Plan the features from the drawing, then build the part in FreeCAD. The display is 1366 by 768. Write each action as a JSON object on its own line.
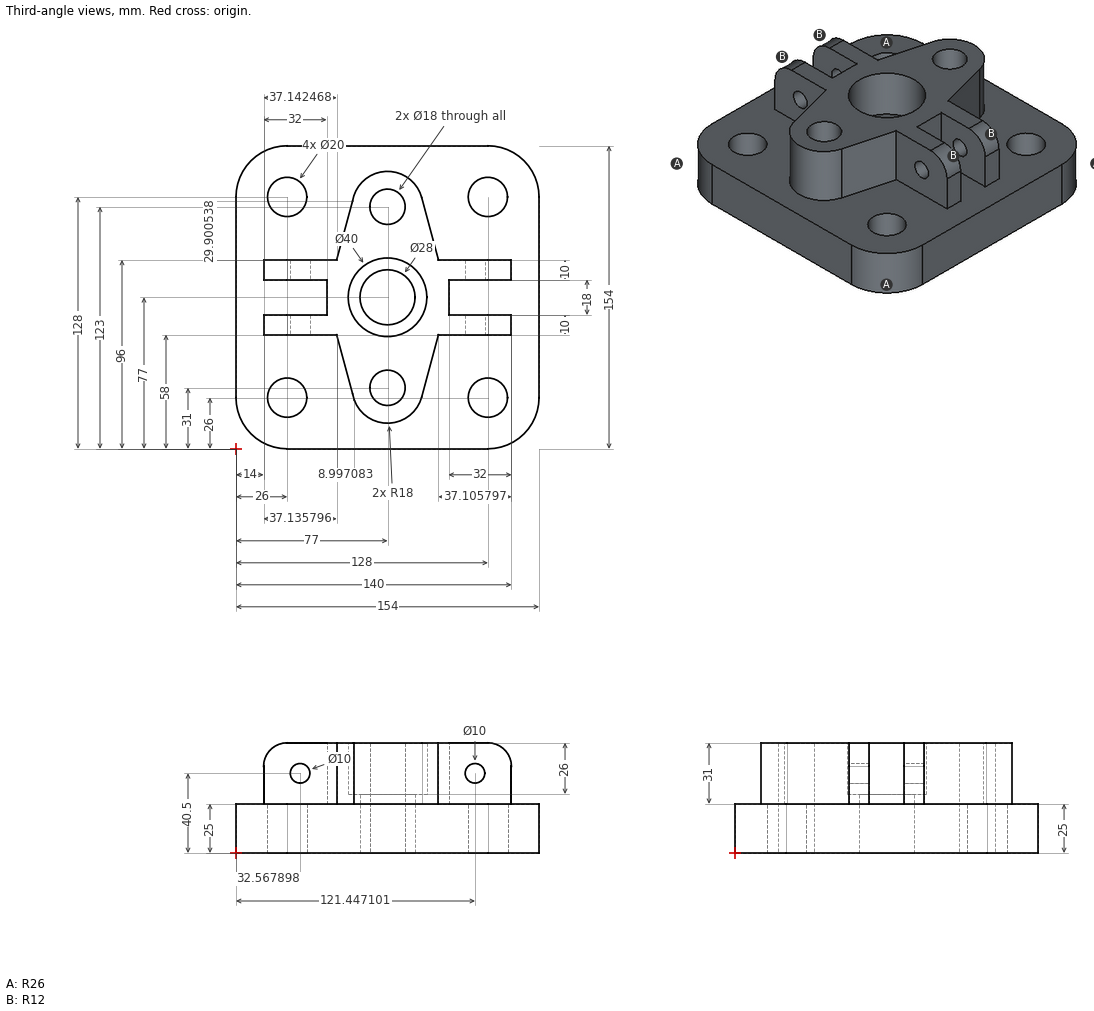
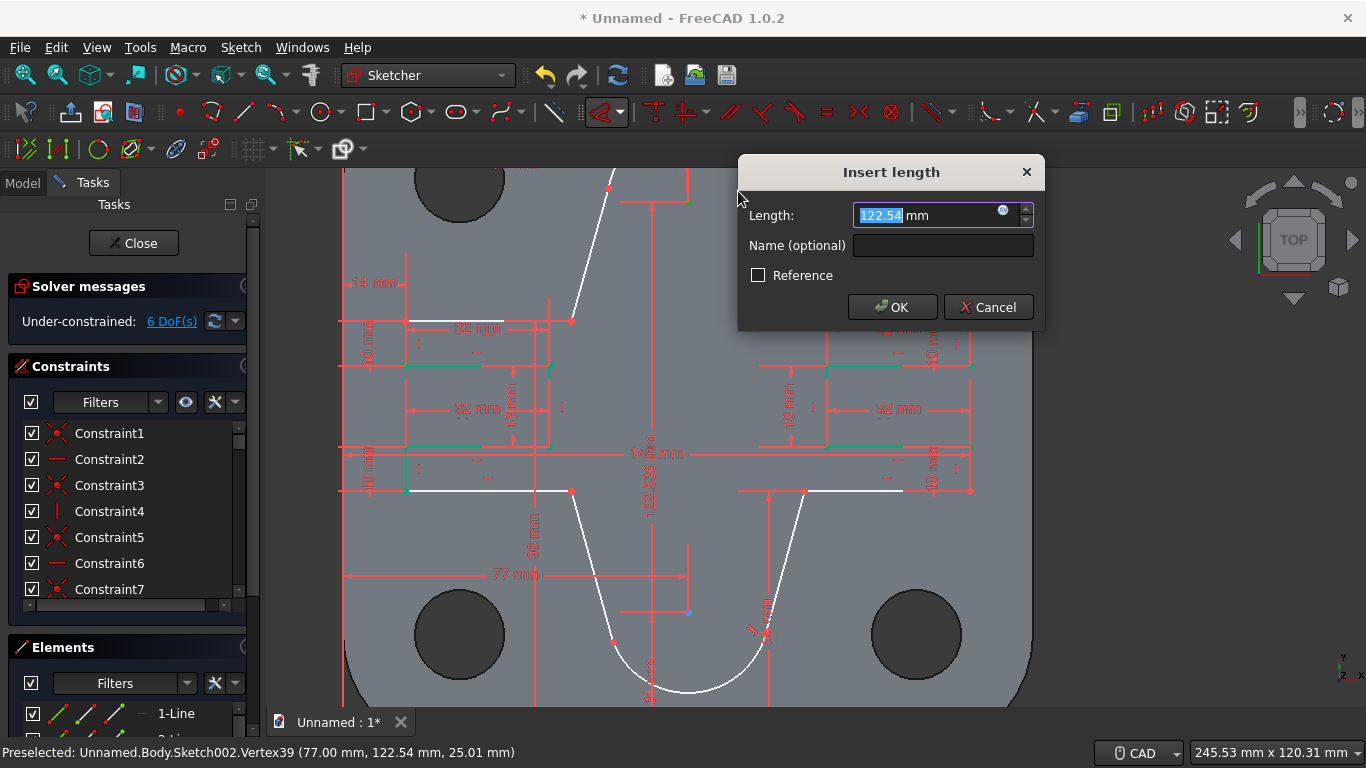
{"action": "type", "text": "123"}
{"action": "key", "text": "Return"}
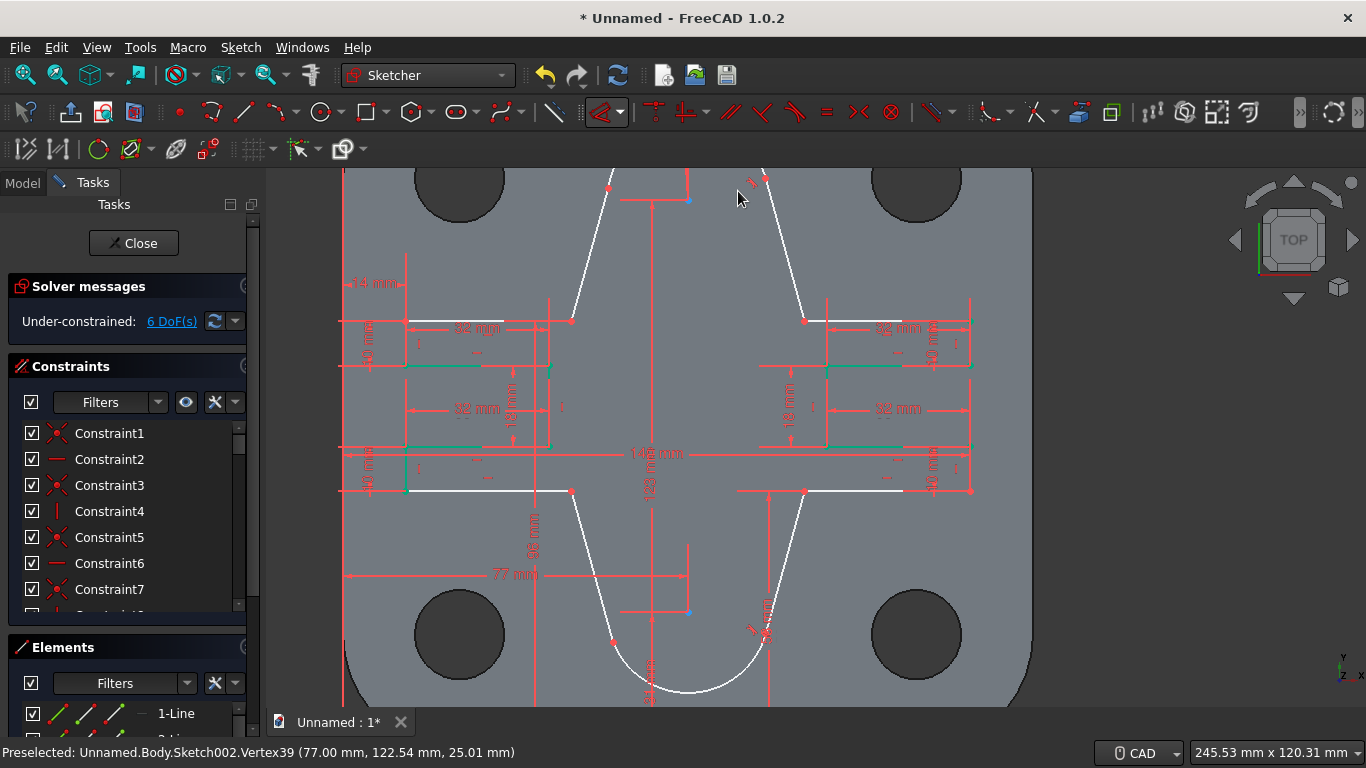
{"action": "left_click", "coordinate": [854, 491]}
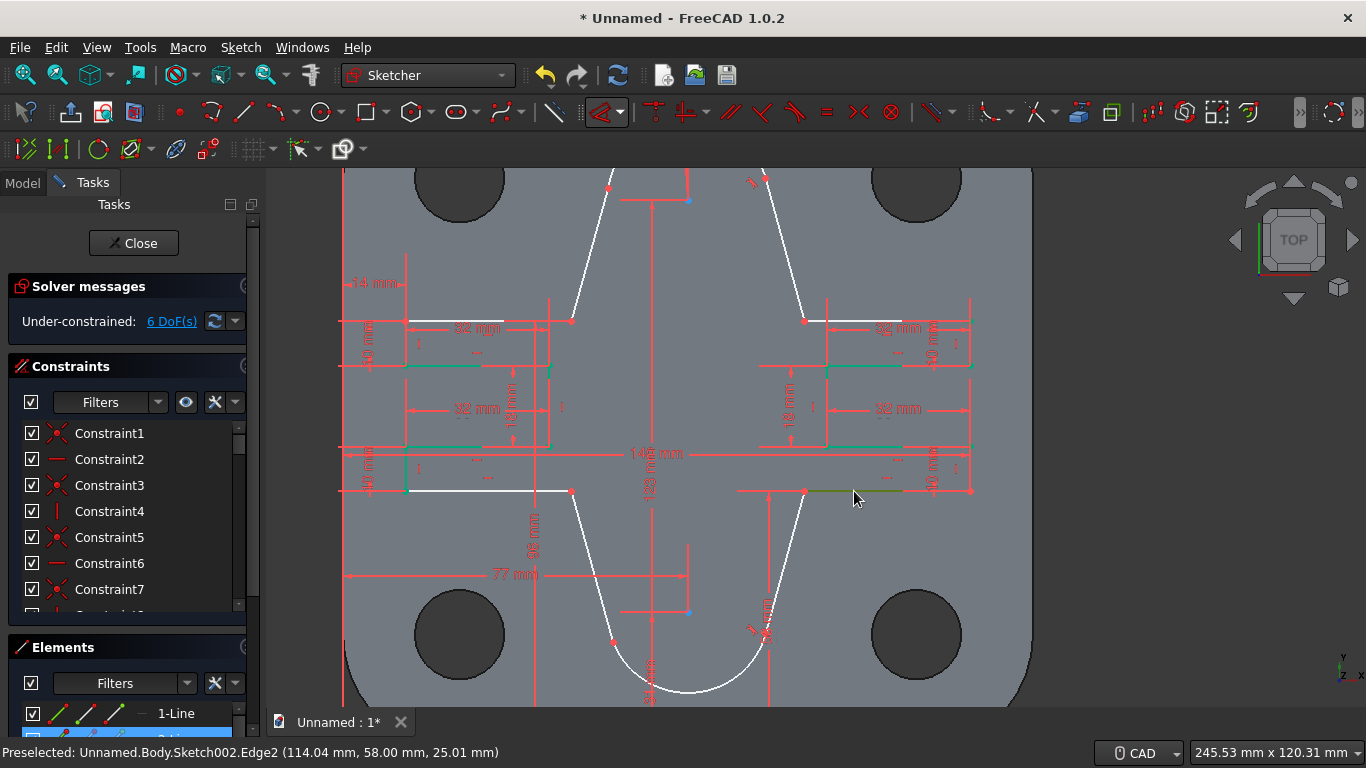
{"action": "left_click", "coordinate": [622, 112]}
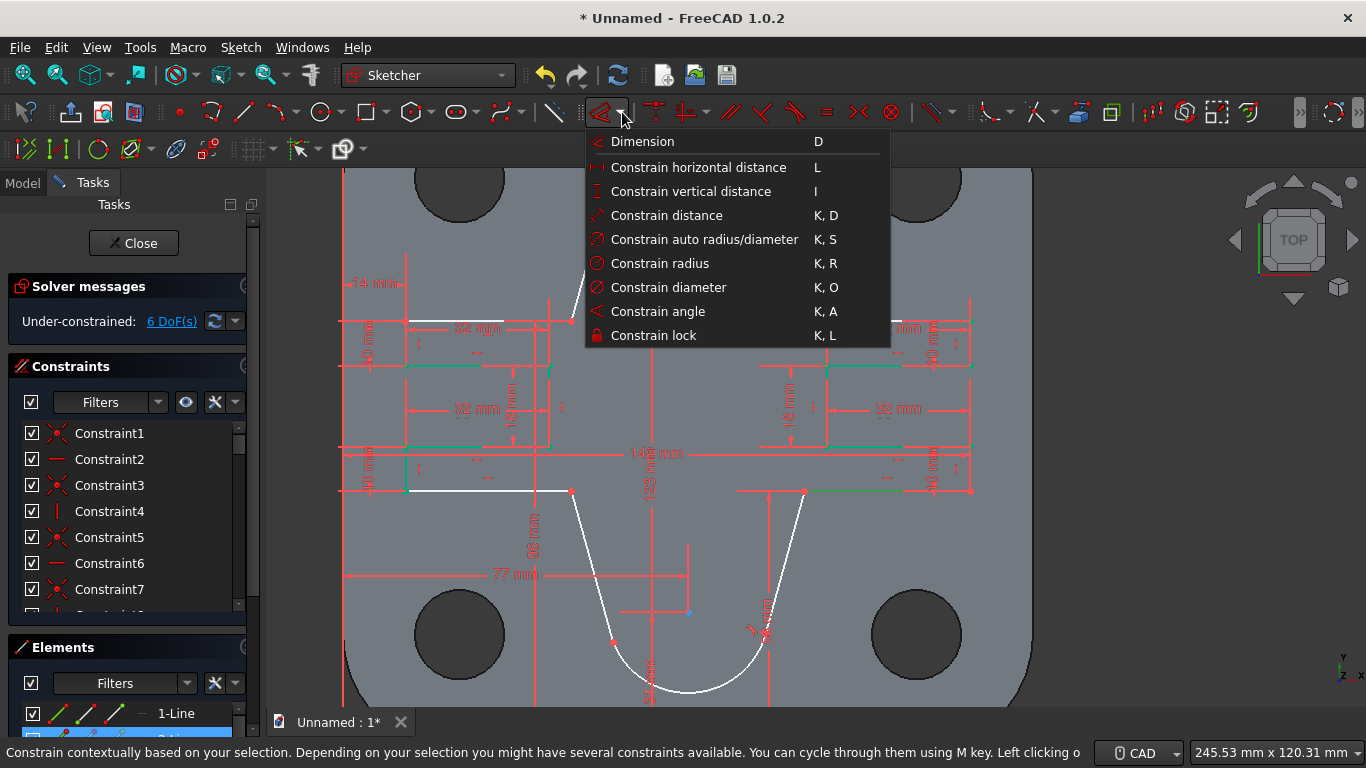
{"action": "left_click", "coordinate": [738, 167]}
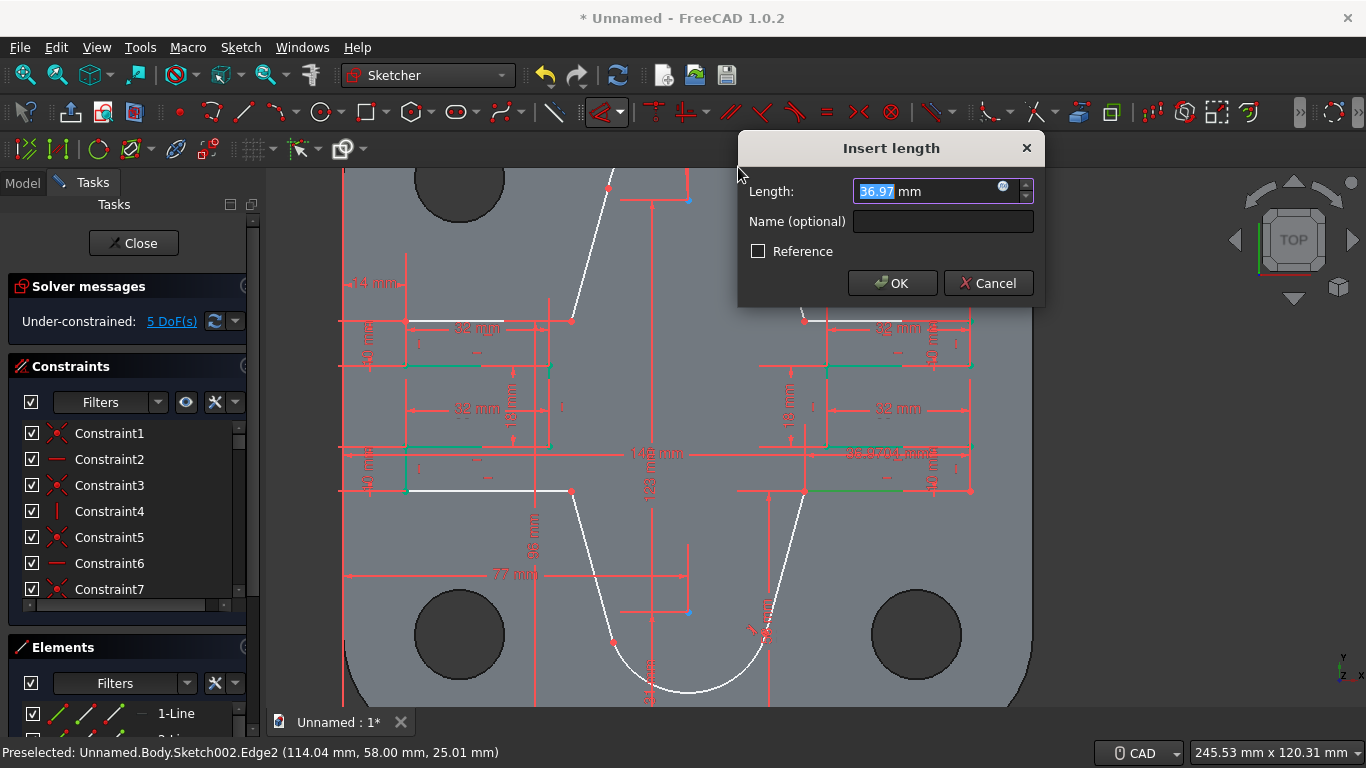
{"action": "type", "text": "37.105797"}
{"action": "key", "text": "Return"}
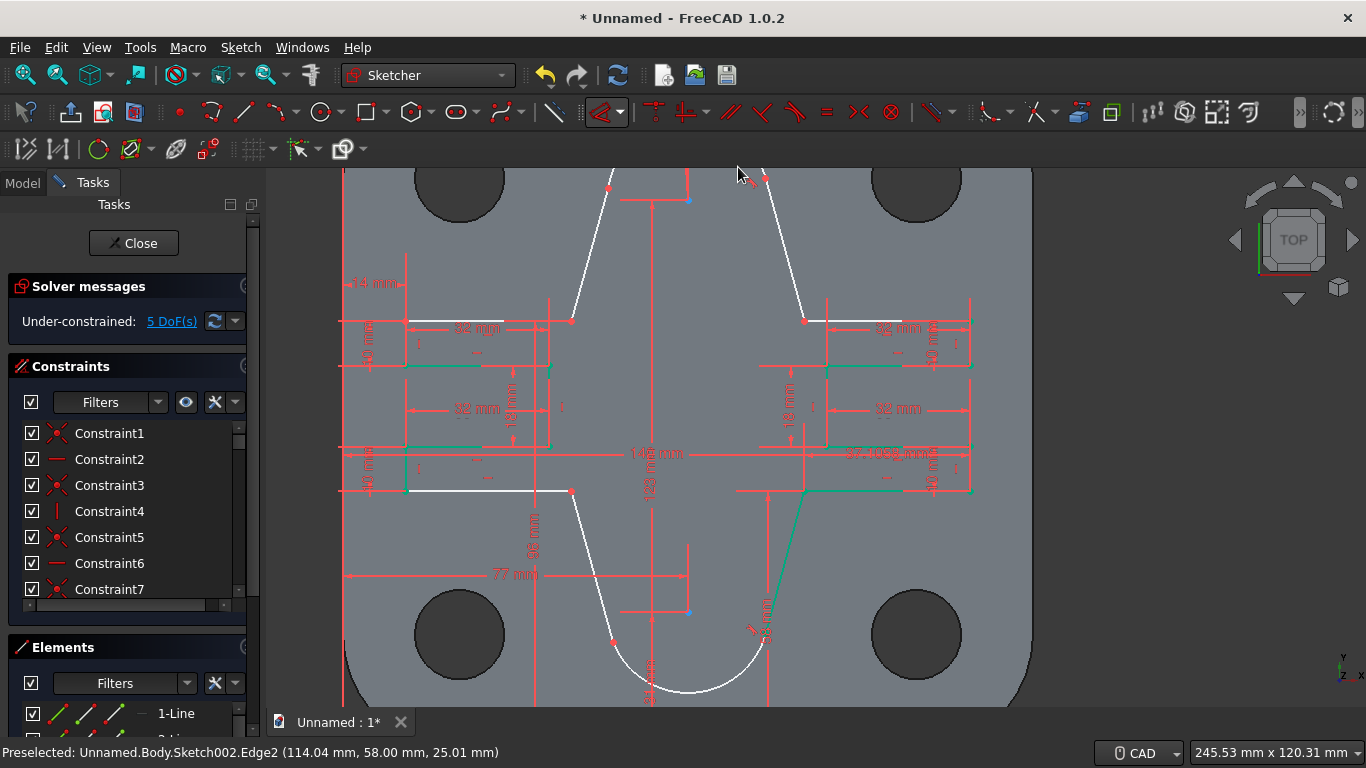
{"action": "left_click", "coordinate": [854, 321]}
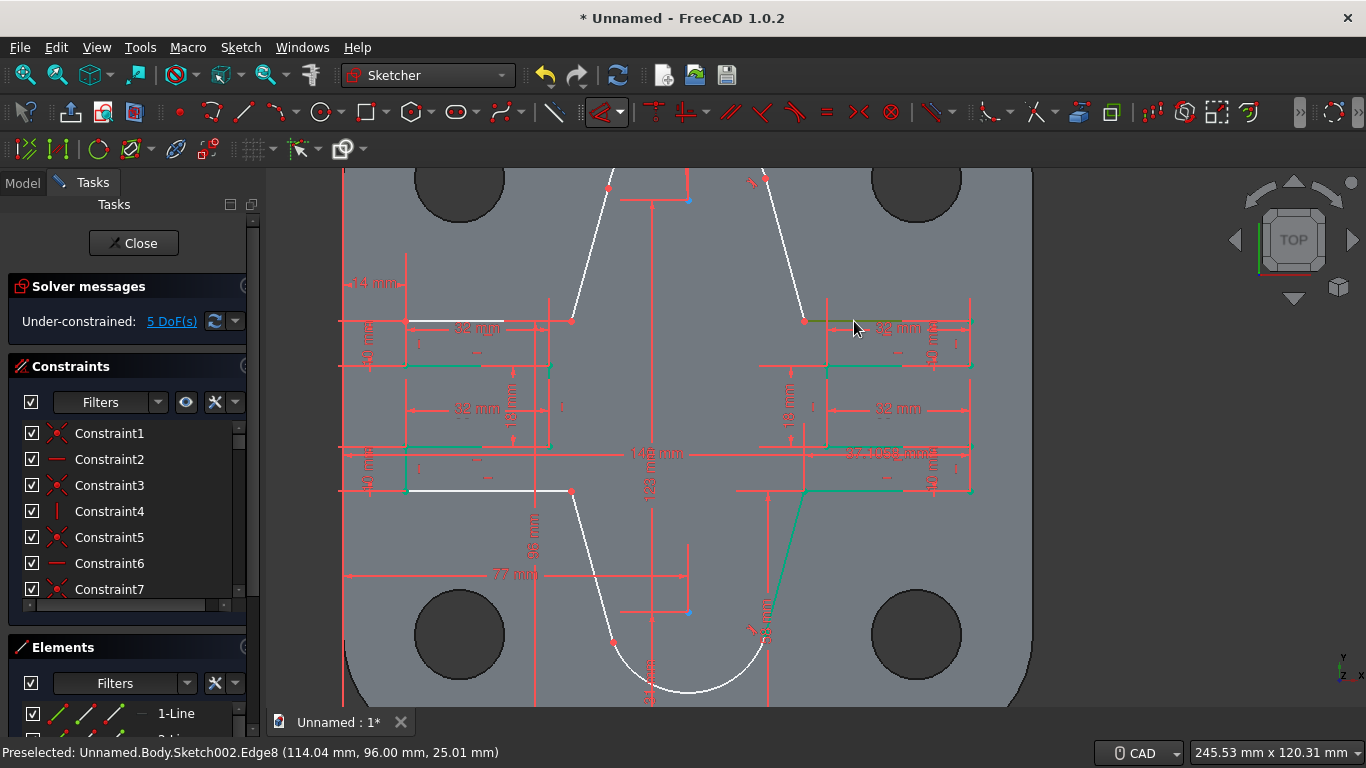
{"action": "key", "text": "l"}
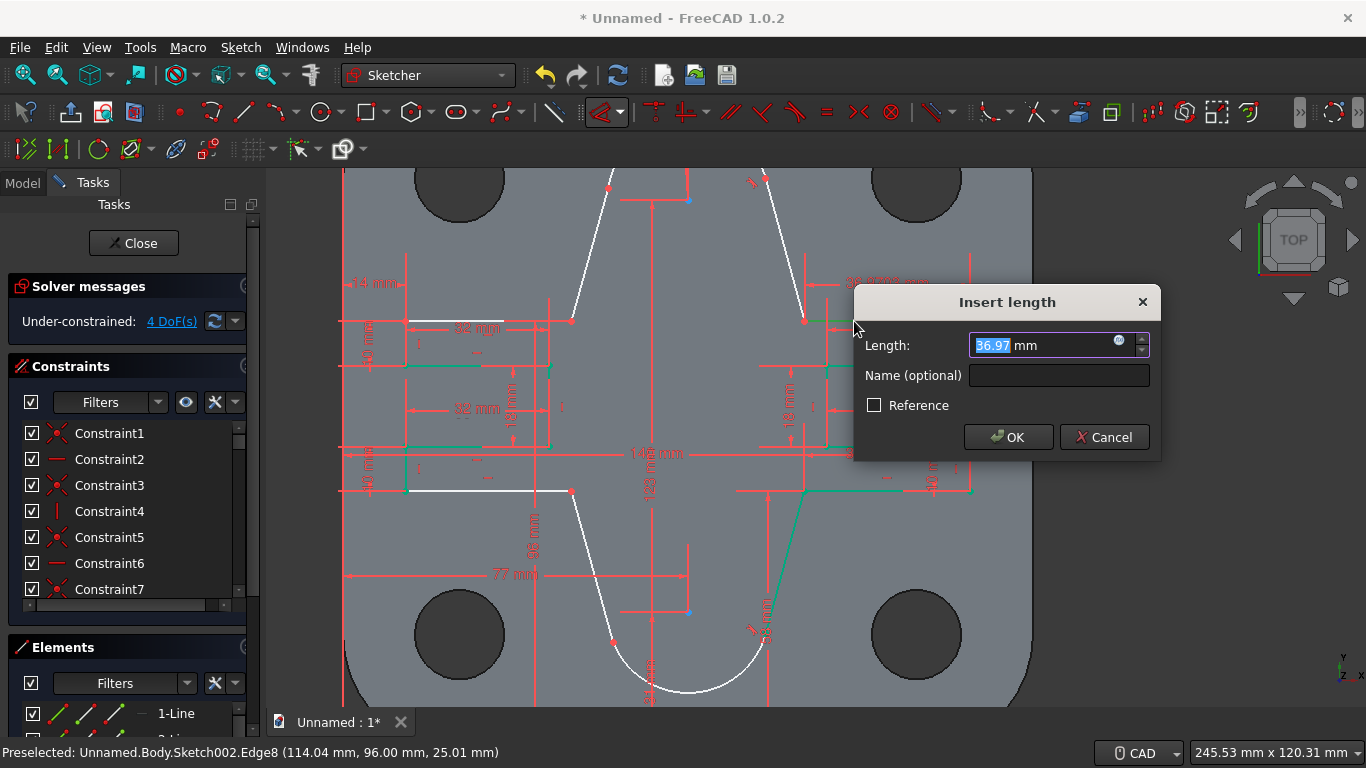
{"action": "type", "text": "37.105797"}
{"action": "key", "text": "Return"}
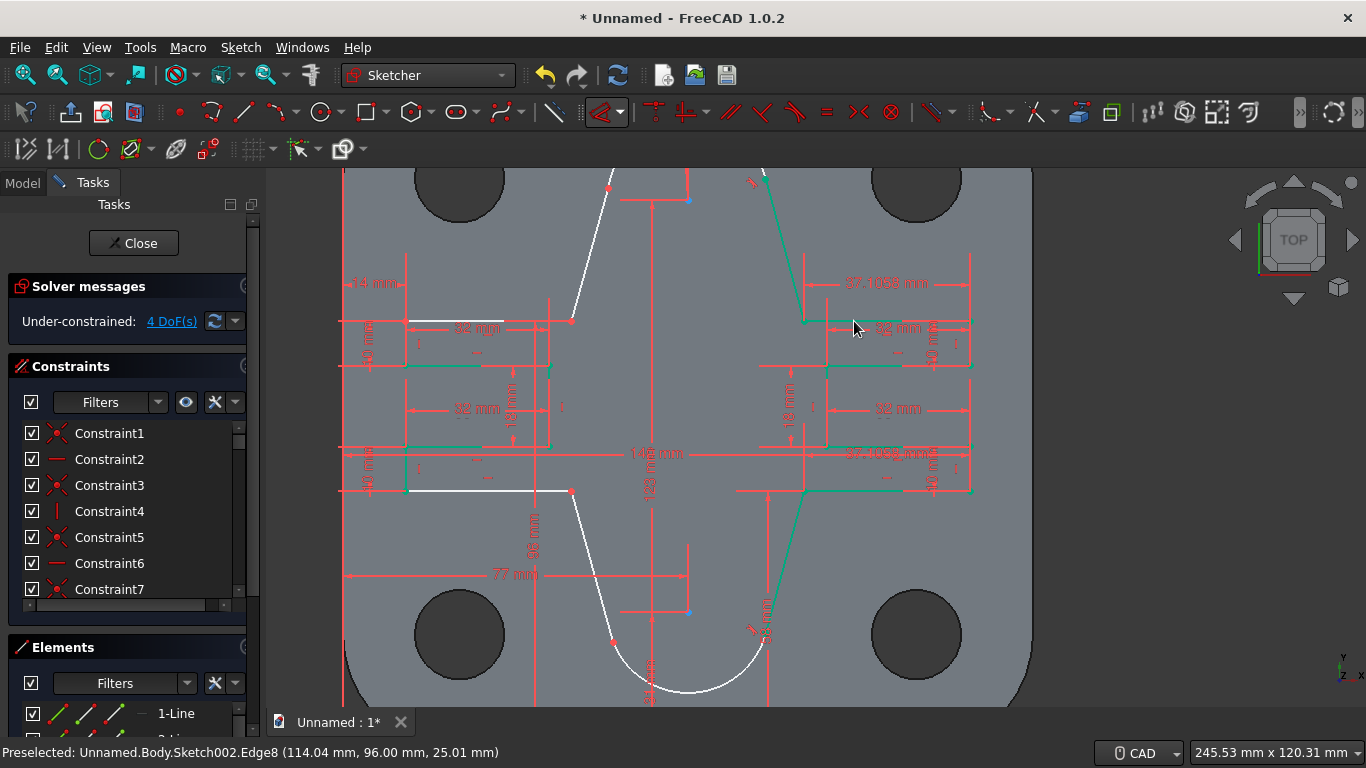
{"action": "left_click", "coordinate": [522, 321]}